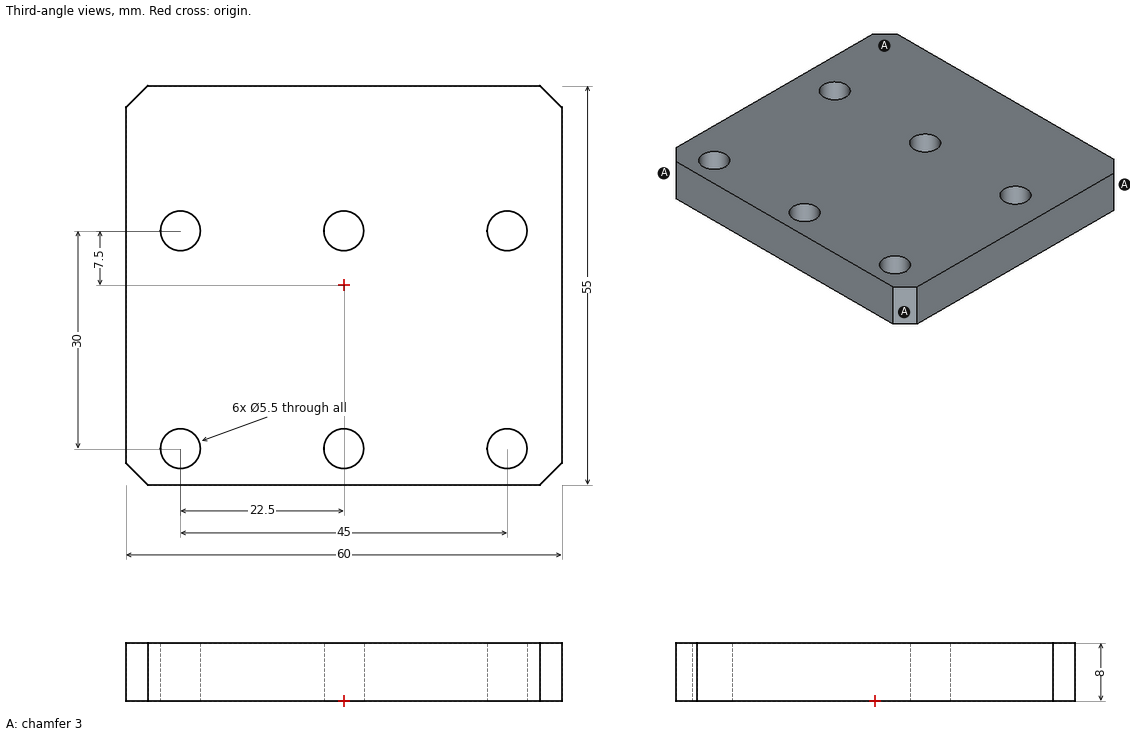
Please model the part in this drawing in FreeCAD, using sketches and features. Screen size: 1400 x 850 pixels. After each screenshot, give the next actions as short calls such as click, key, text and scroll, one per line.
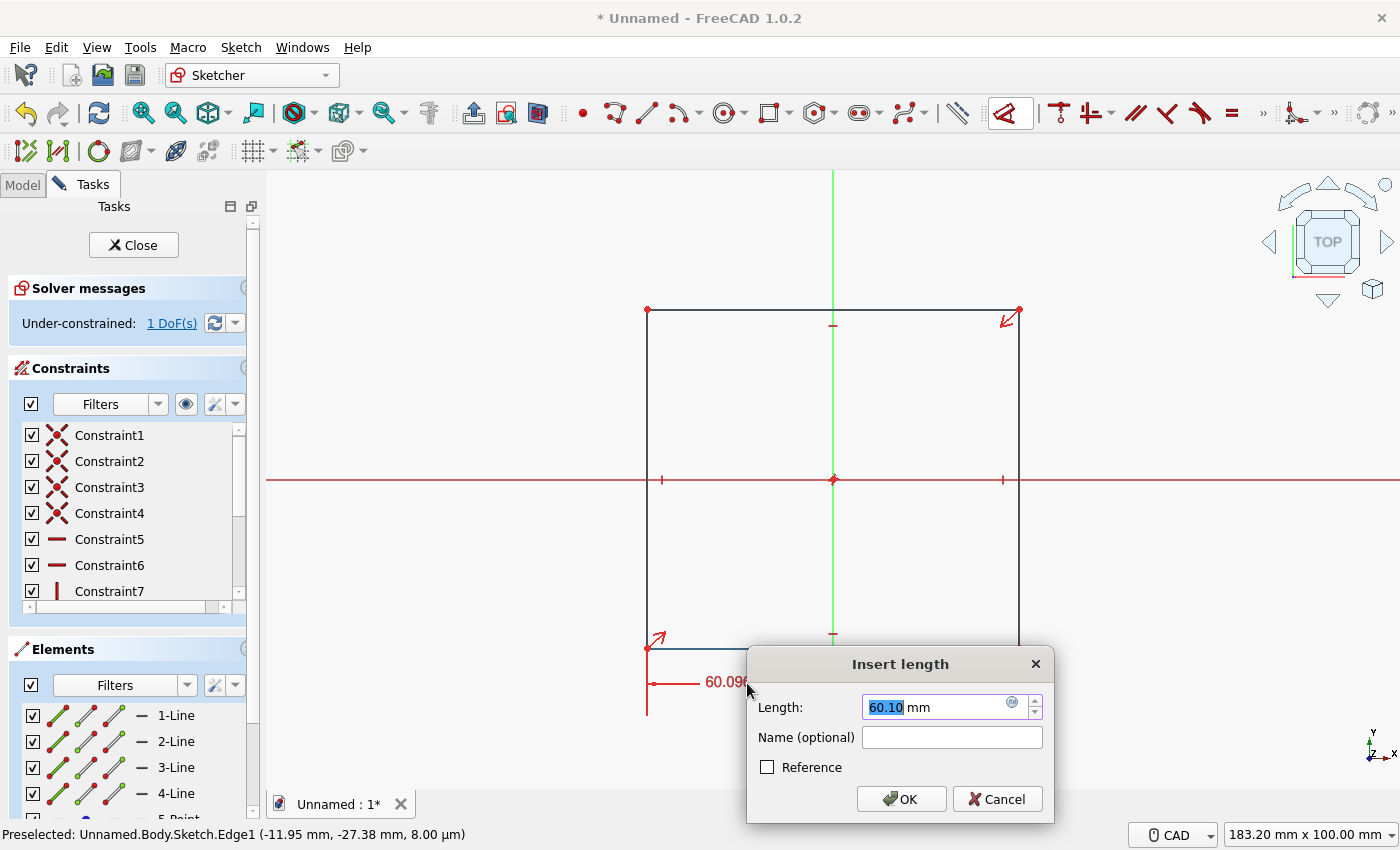
text(60)
key(Return)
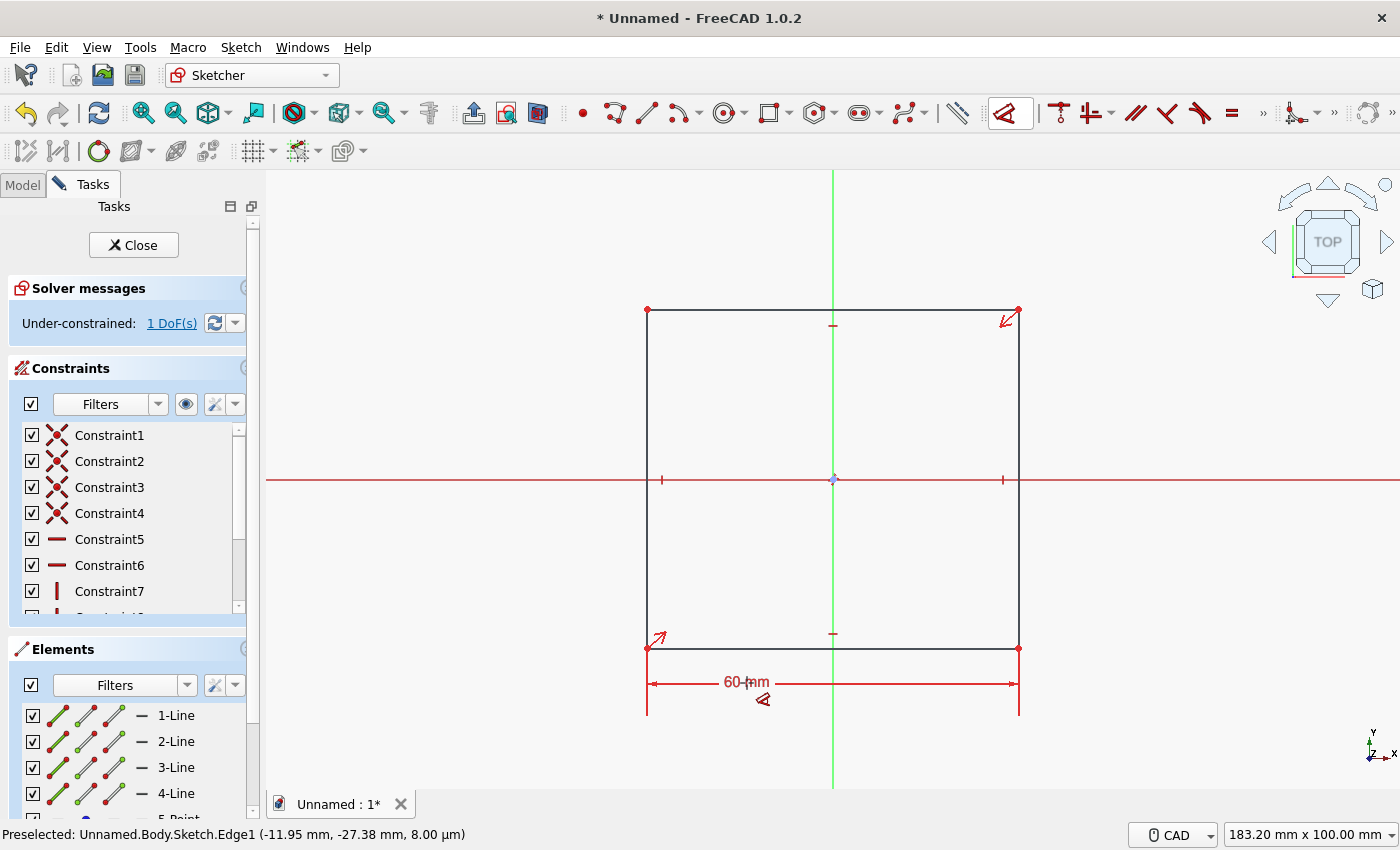
click(1019, 547)
click(1053, 402)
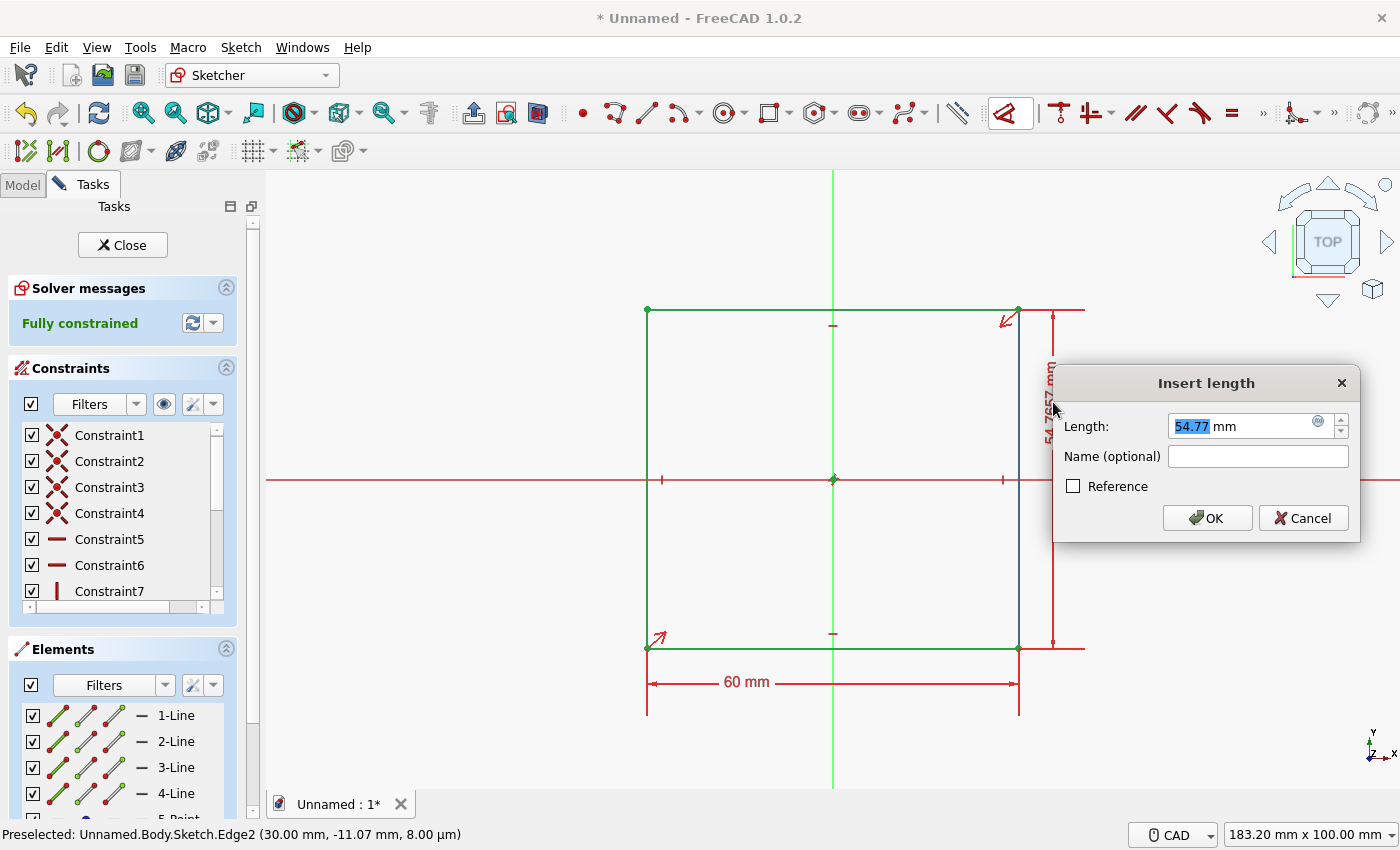
text(55)
key(Return)
key(Escape)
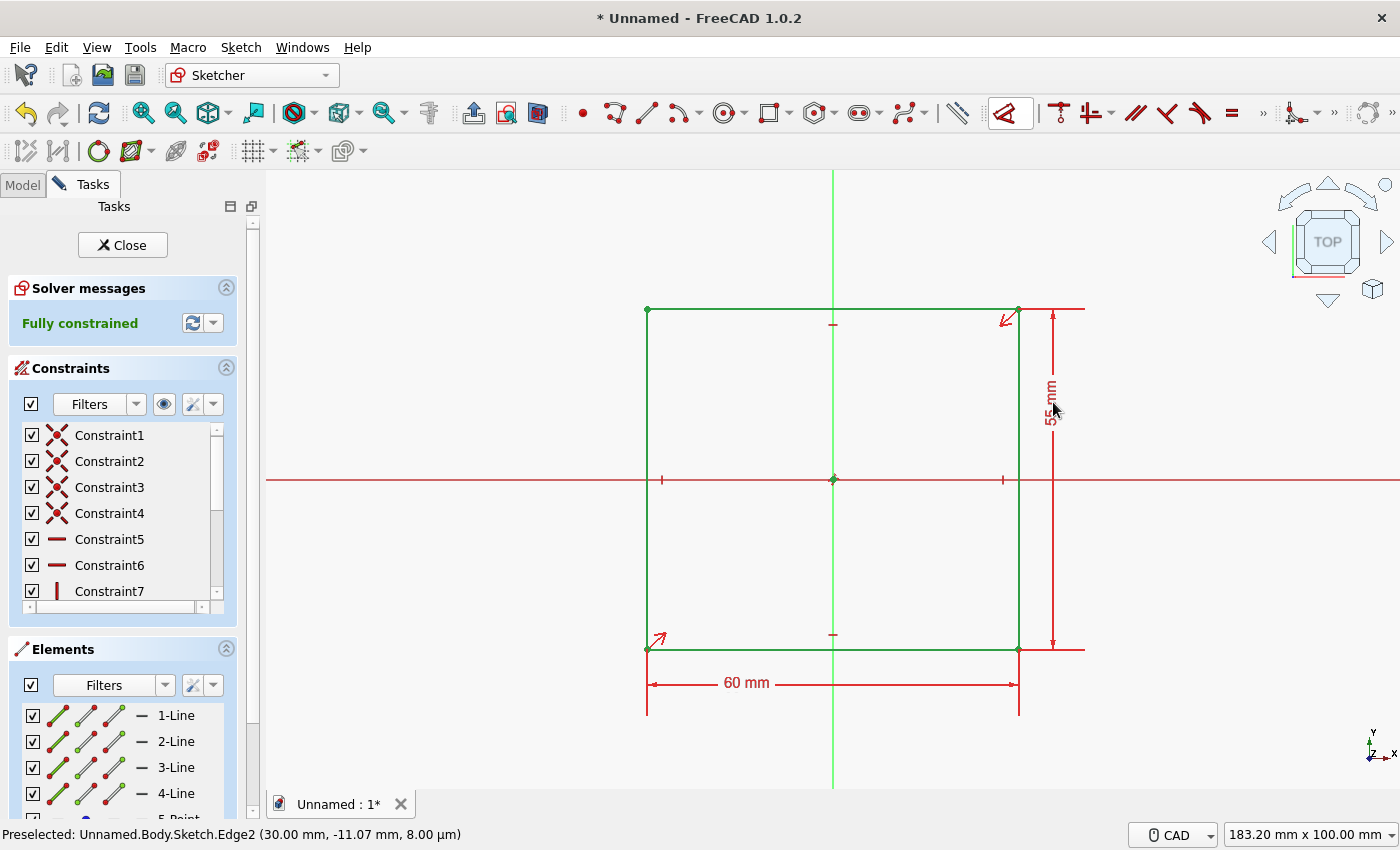
click(123, 245)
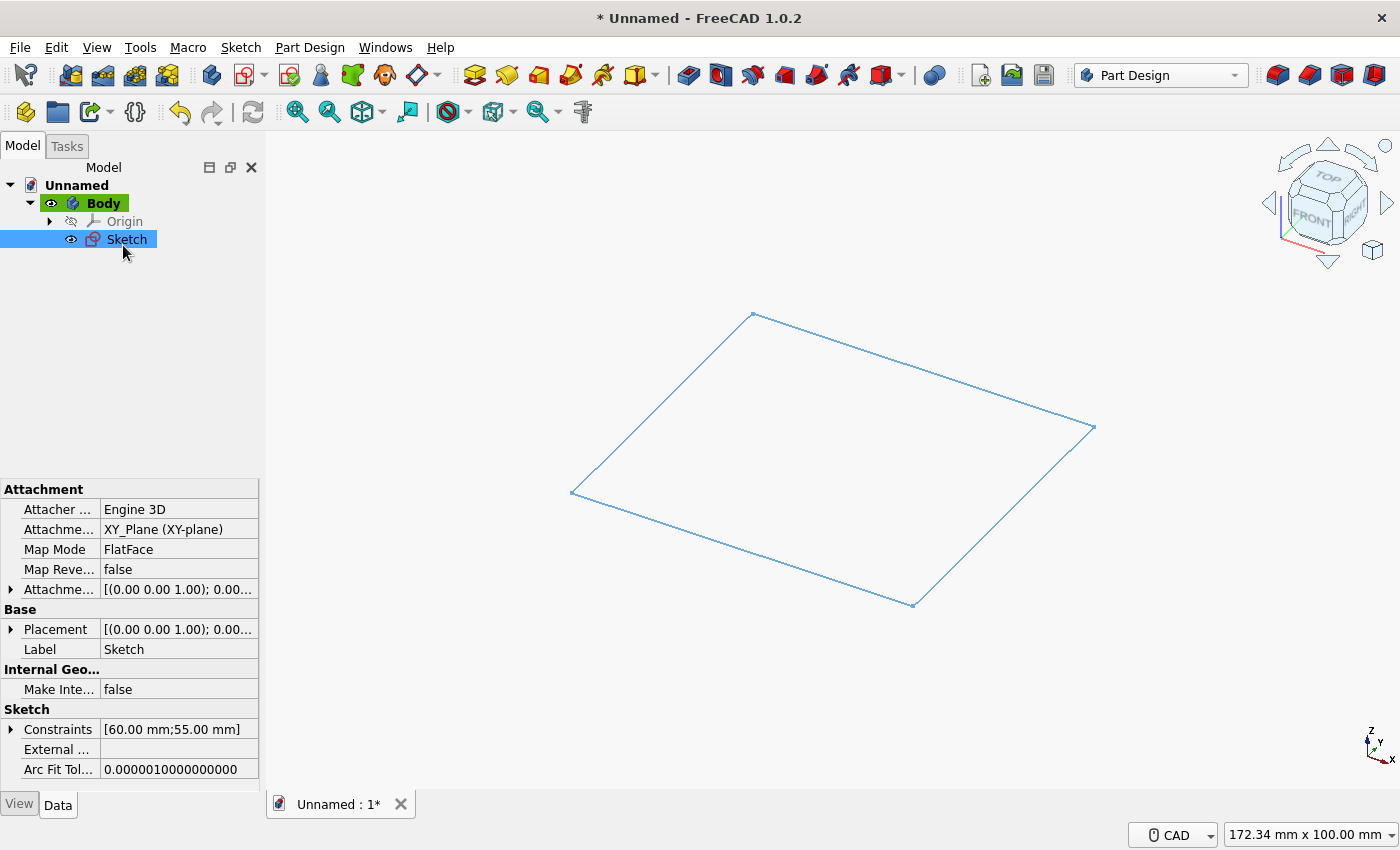
click(476, 76)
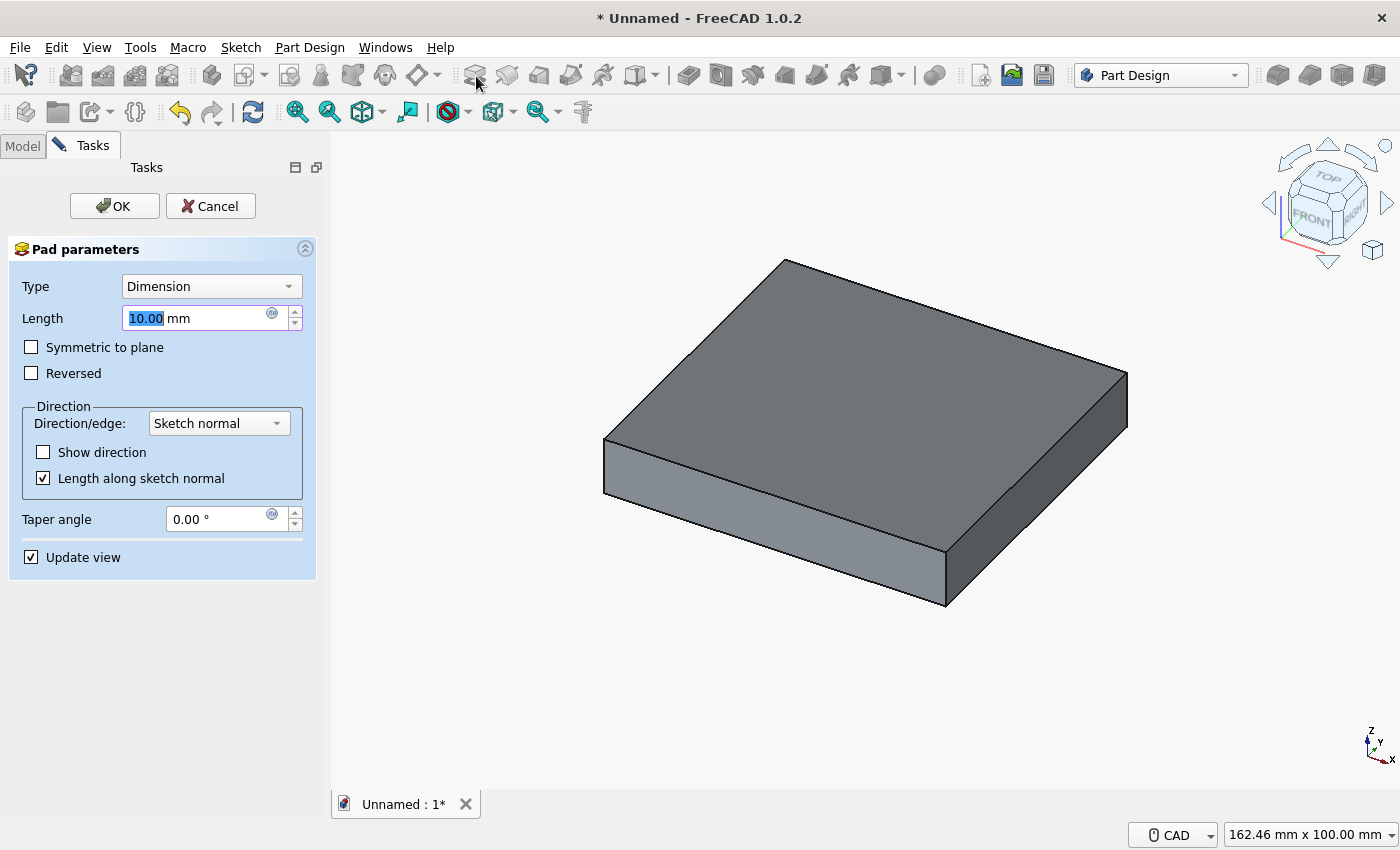
text(8)
key(Tab)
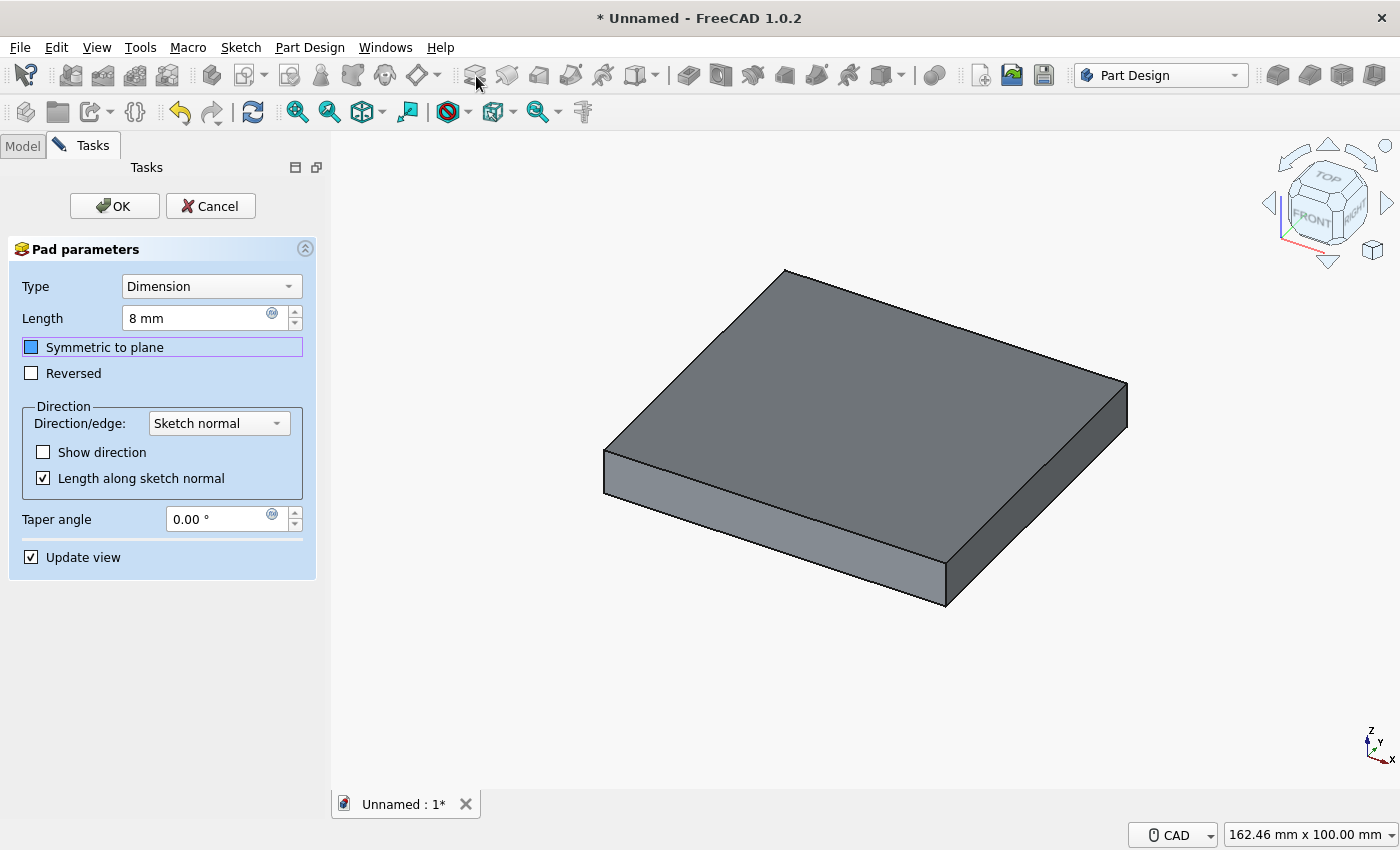
click(115, 206)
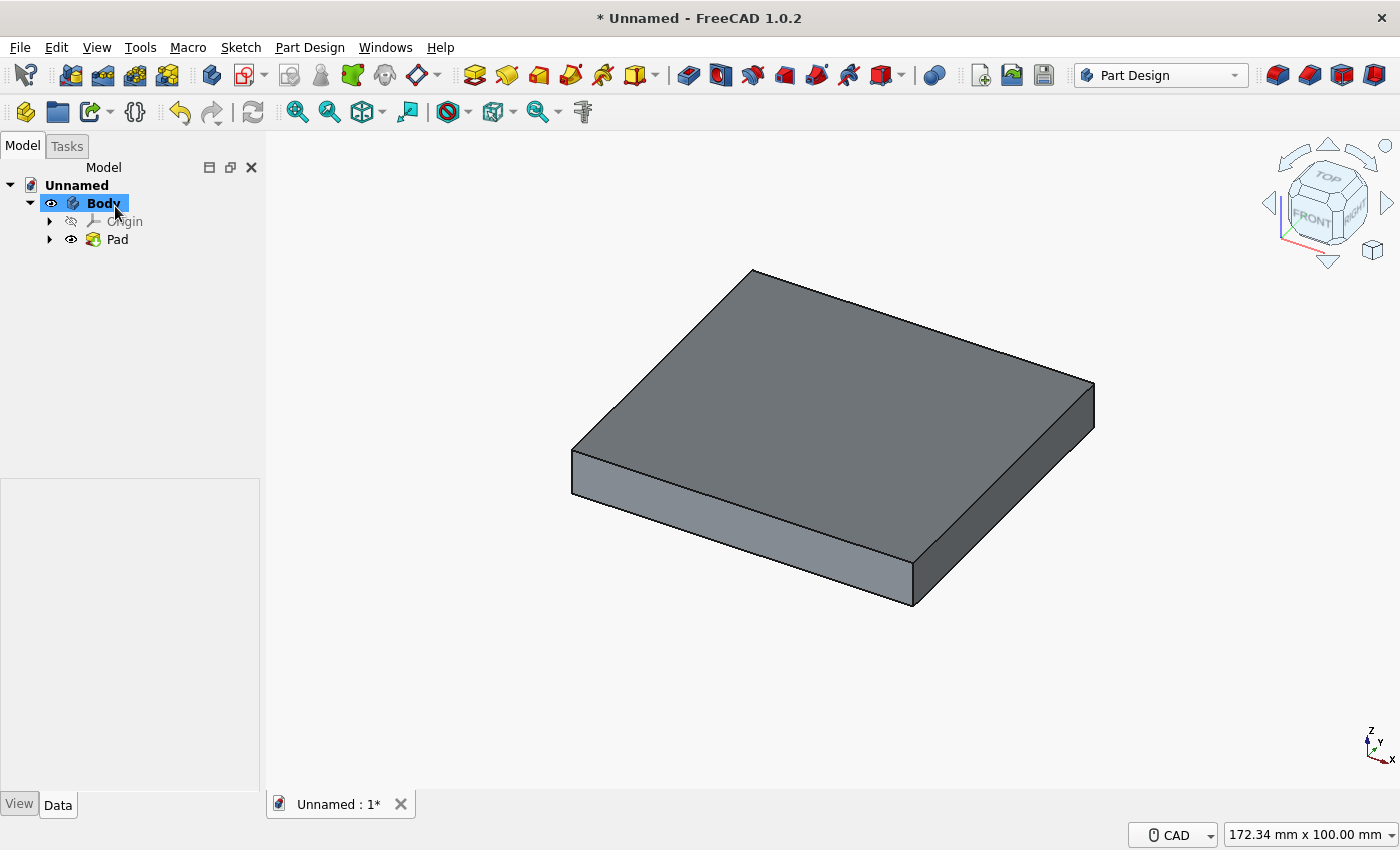
click(833, 416)